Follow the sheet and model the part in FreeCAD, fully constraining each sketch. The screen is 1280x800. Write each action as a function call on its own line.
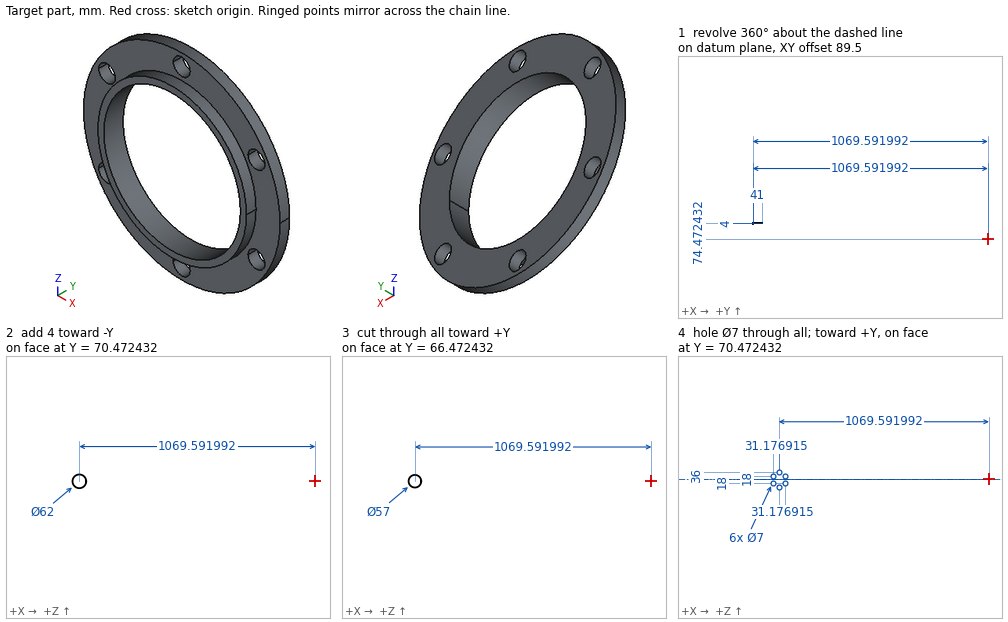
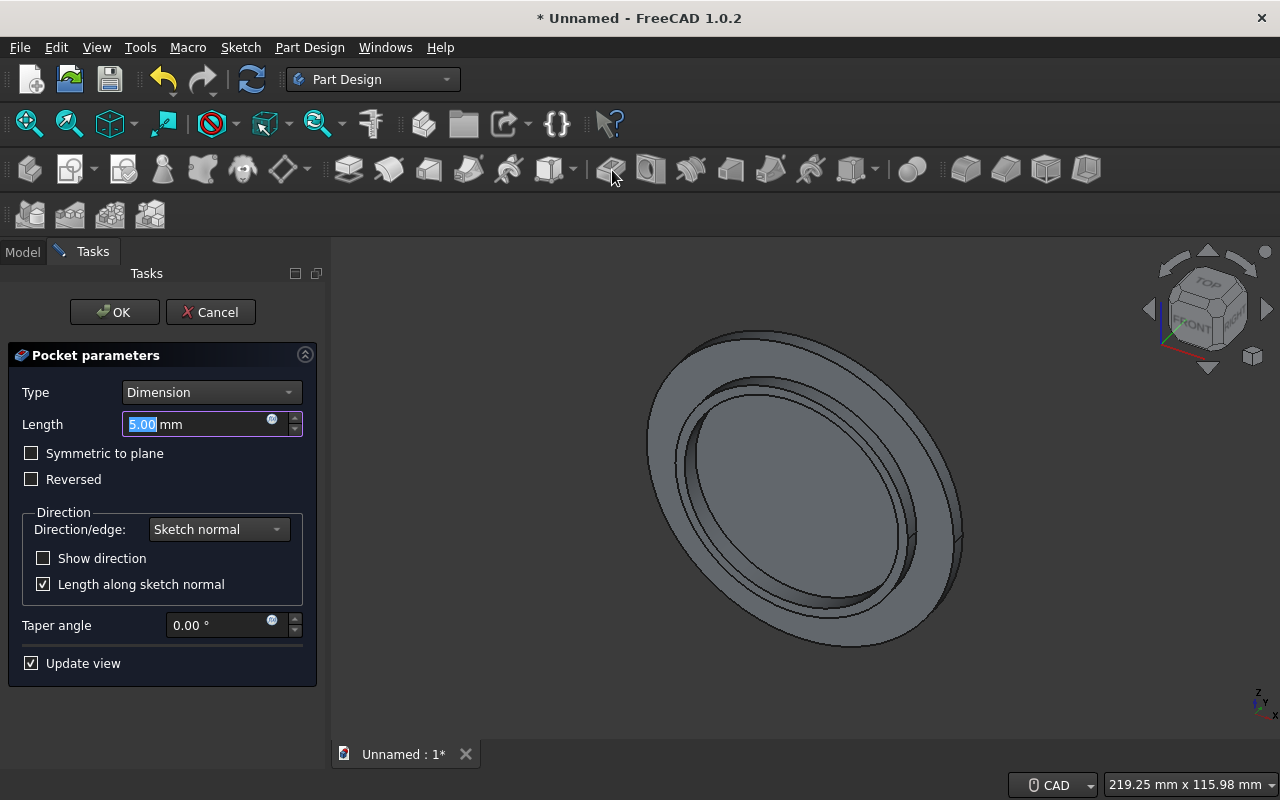
click(212, 392)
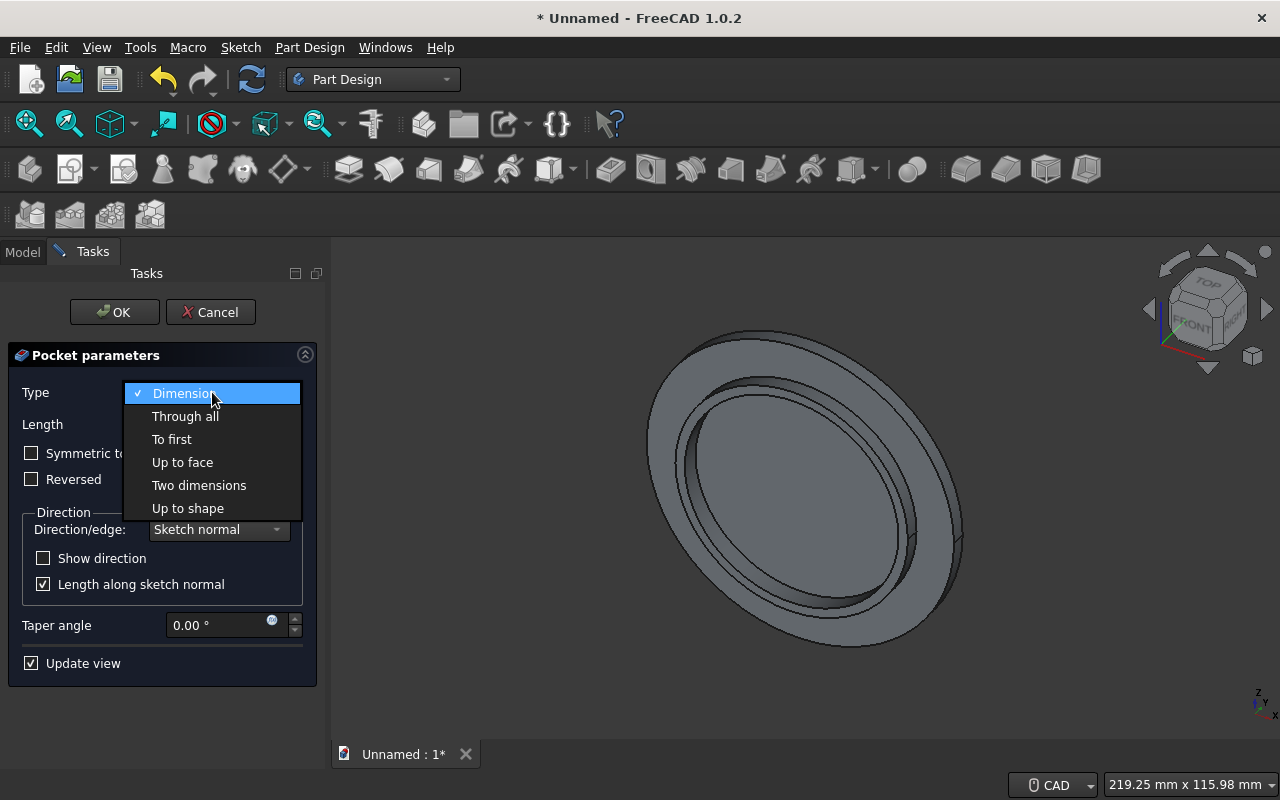
click(212, 416)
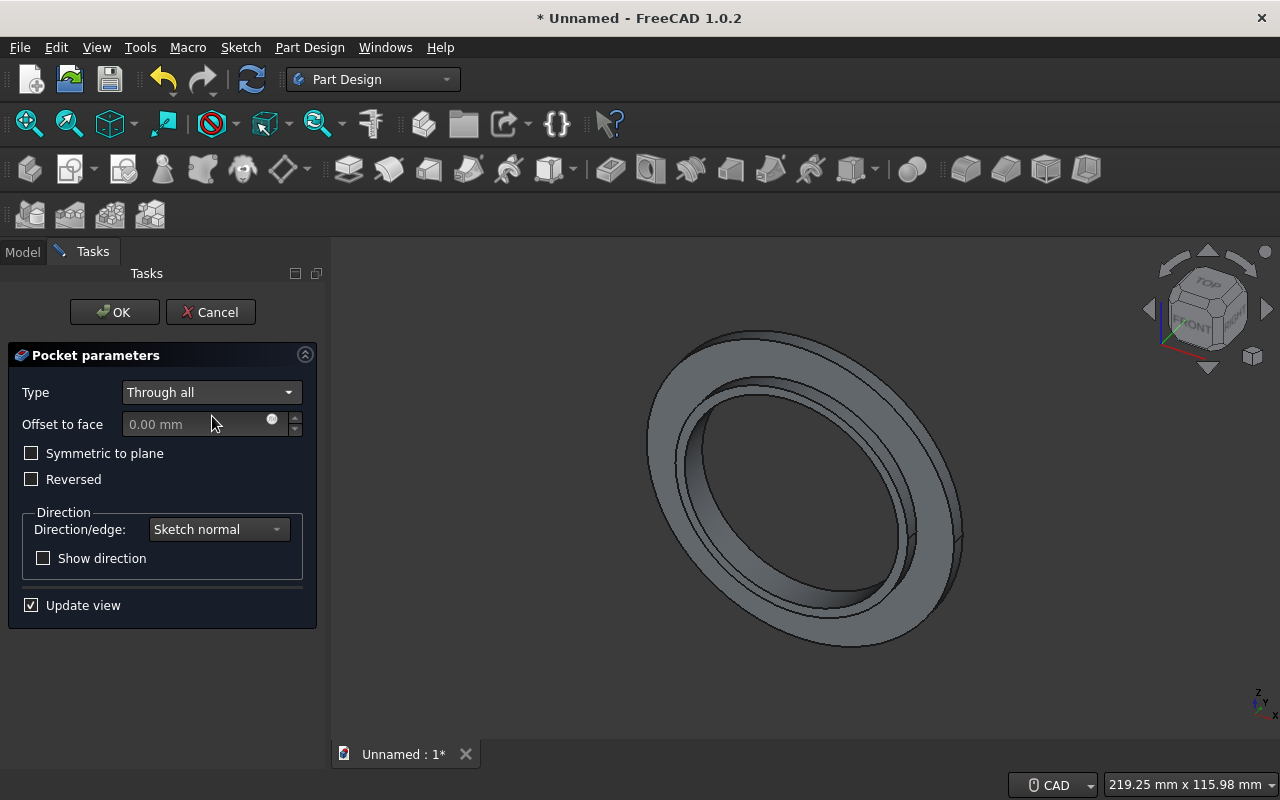
click(115, 312)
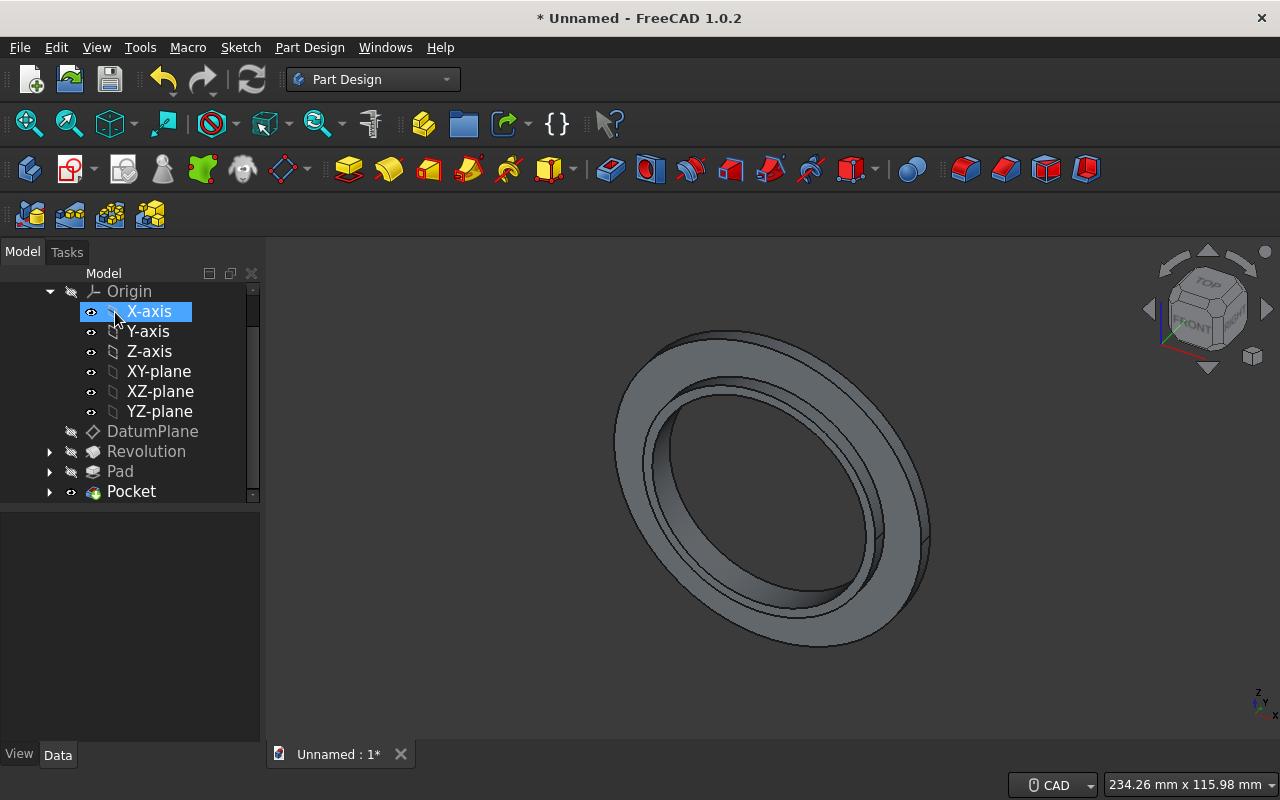
click(768, 367)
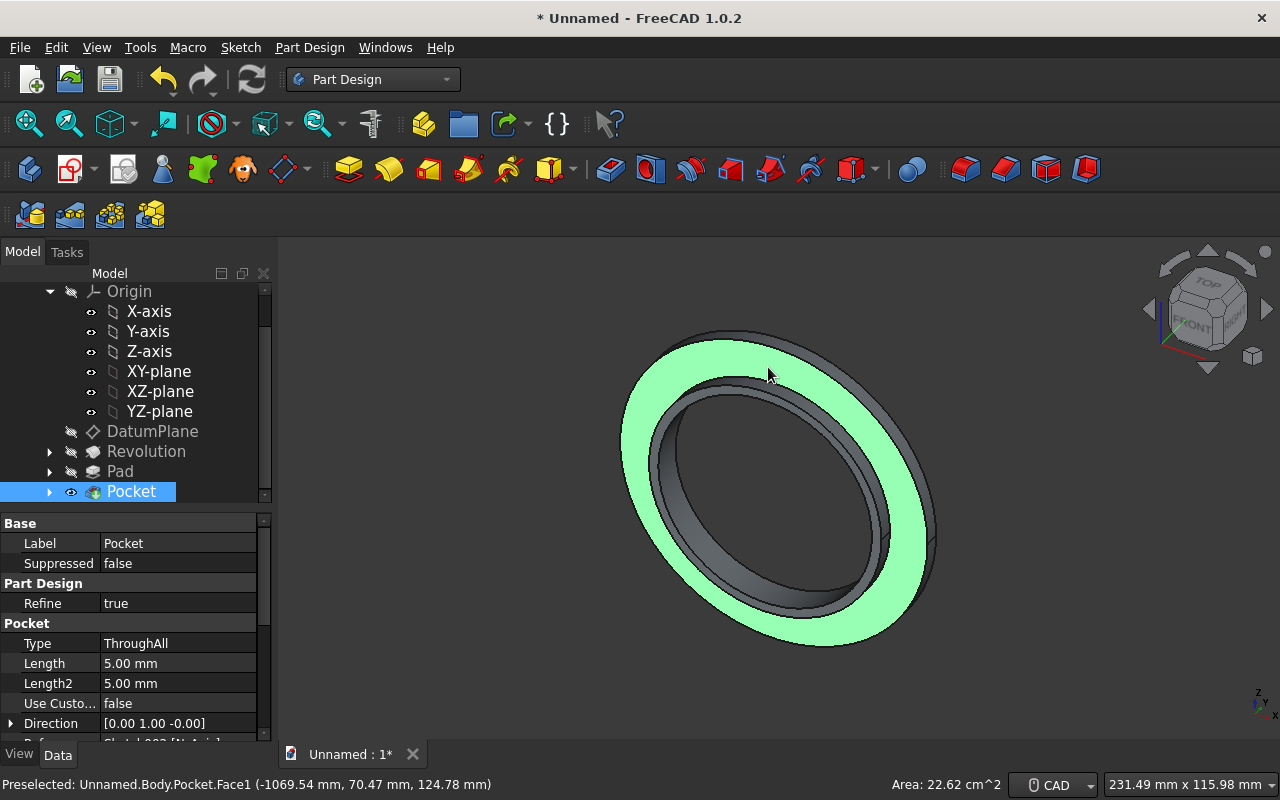
click(70, 170)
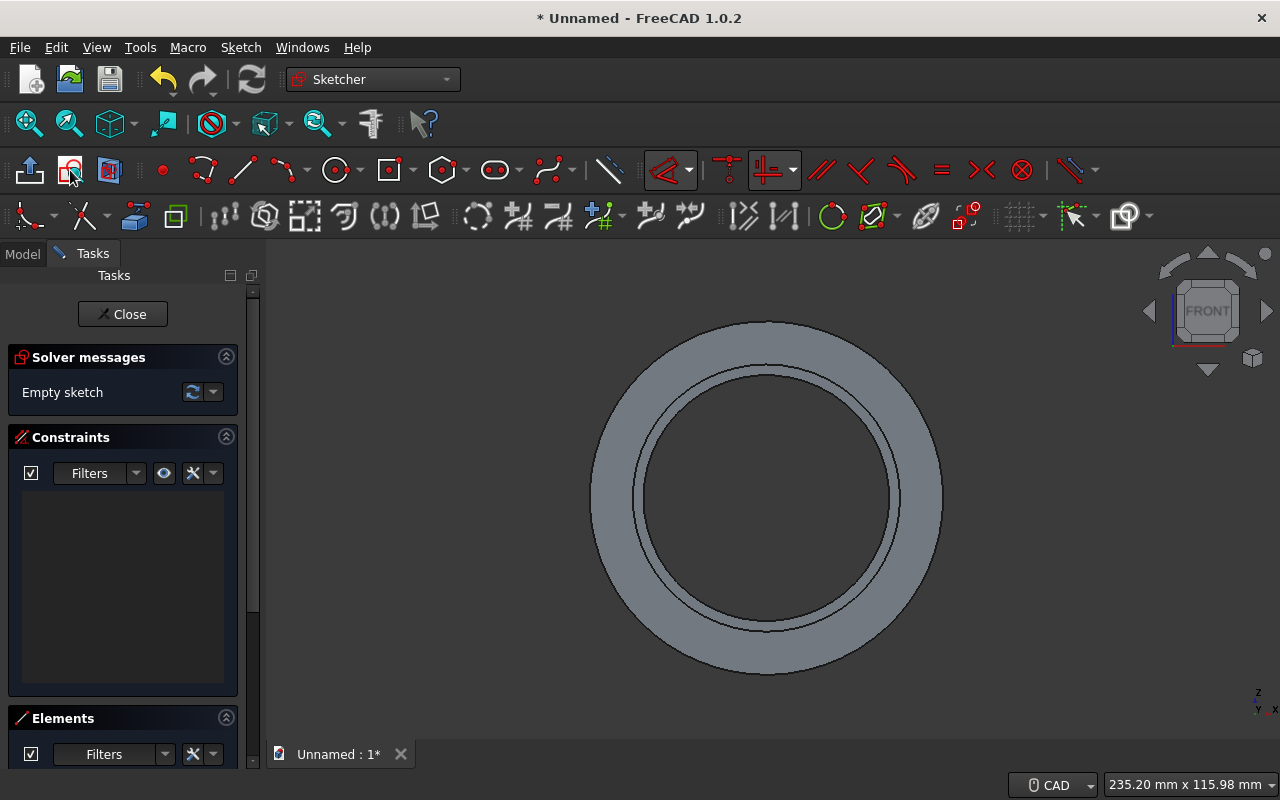
click(110, 170)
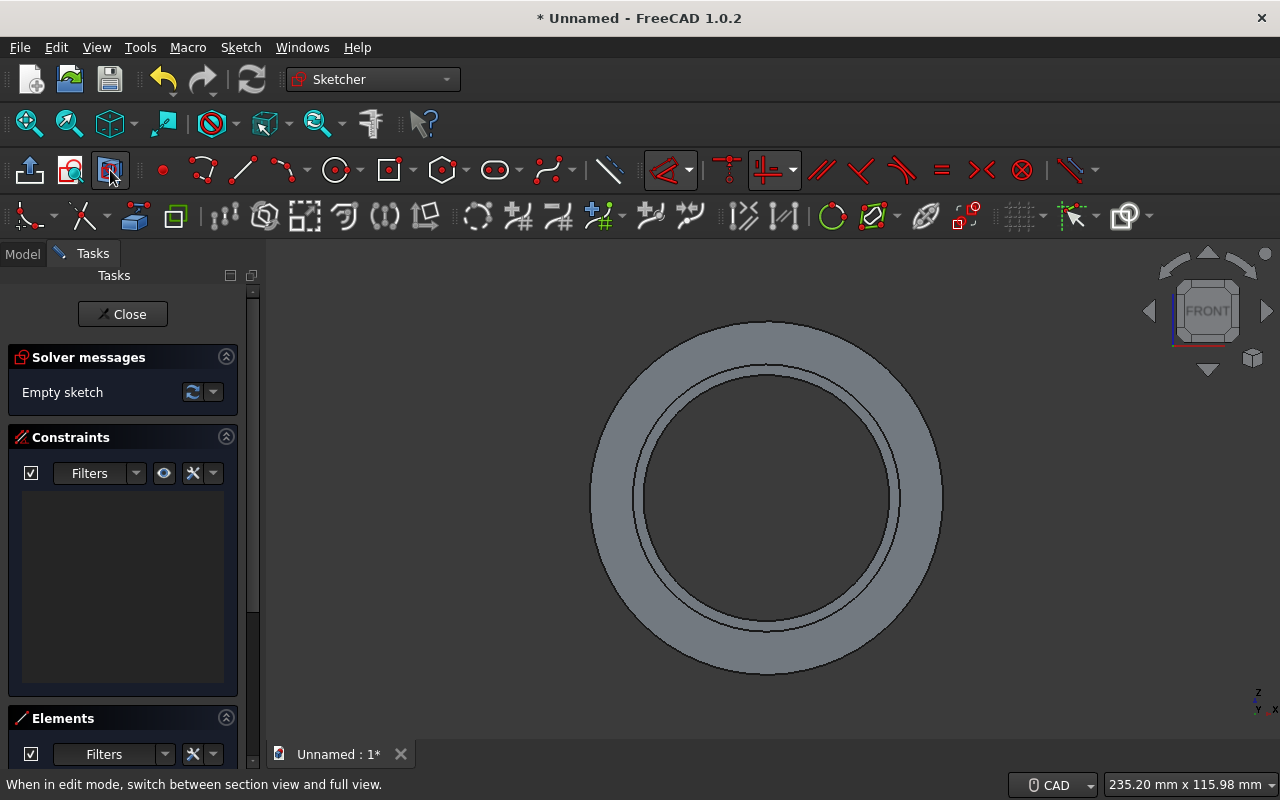
click(336, 170)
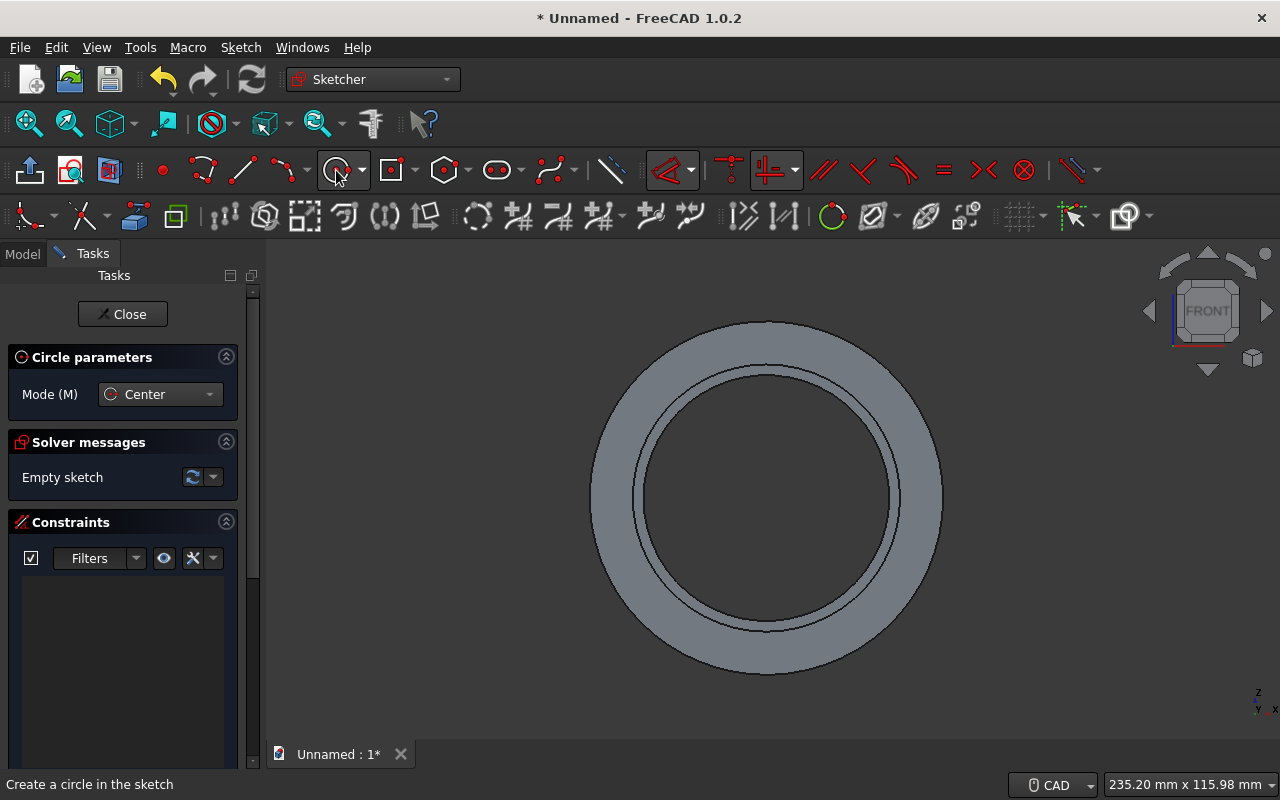
scroll(766, 343, up, 3)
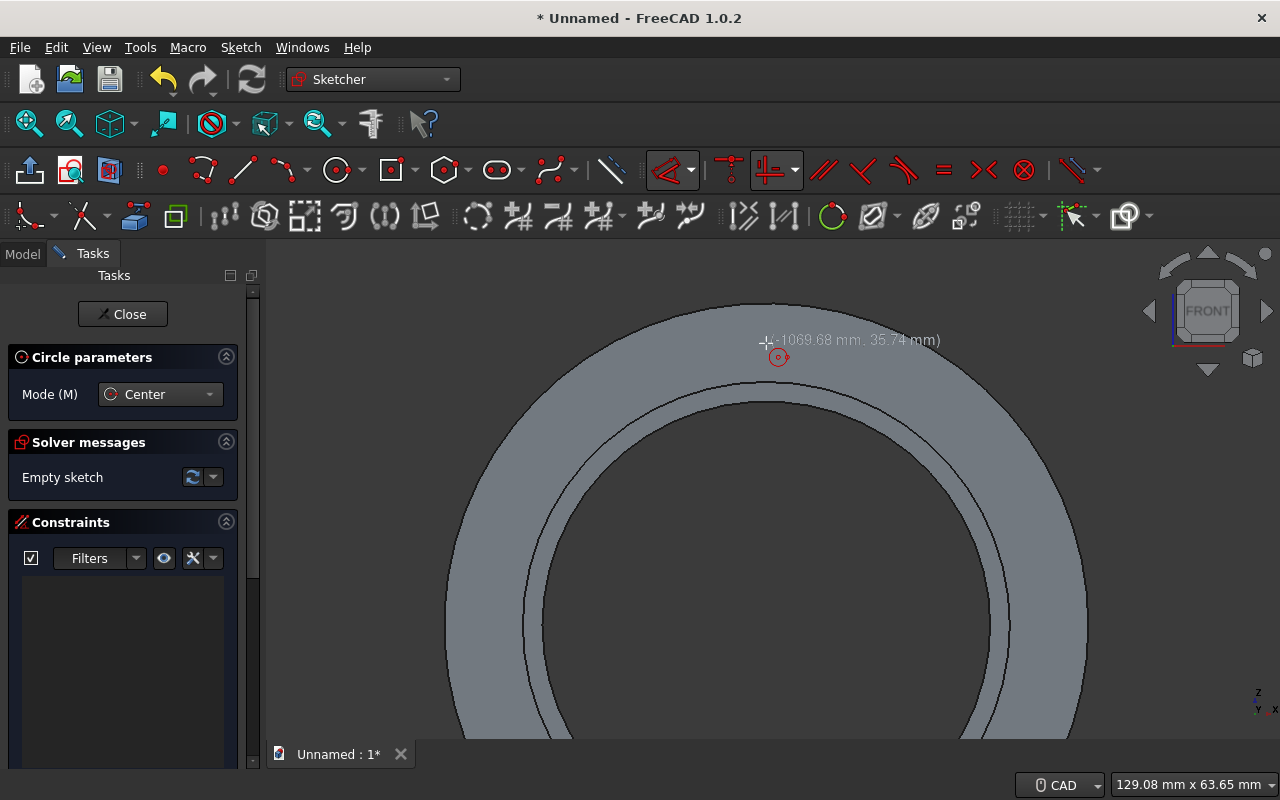
click(766, 343)
move(786, 323)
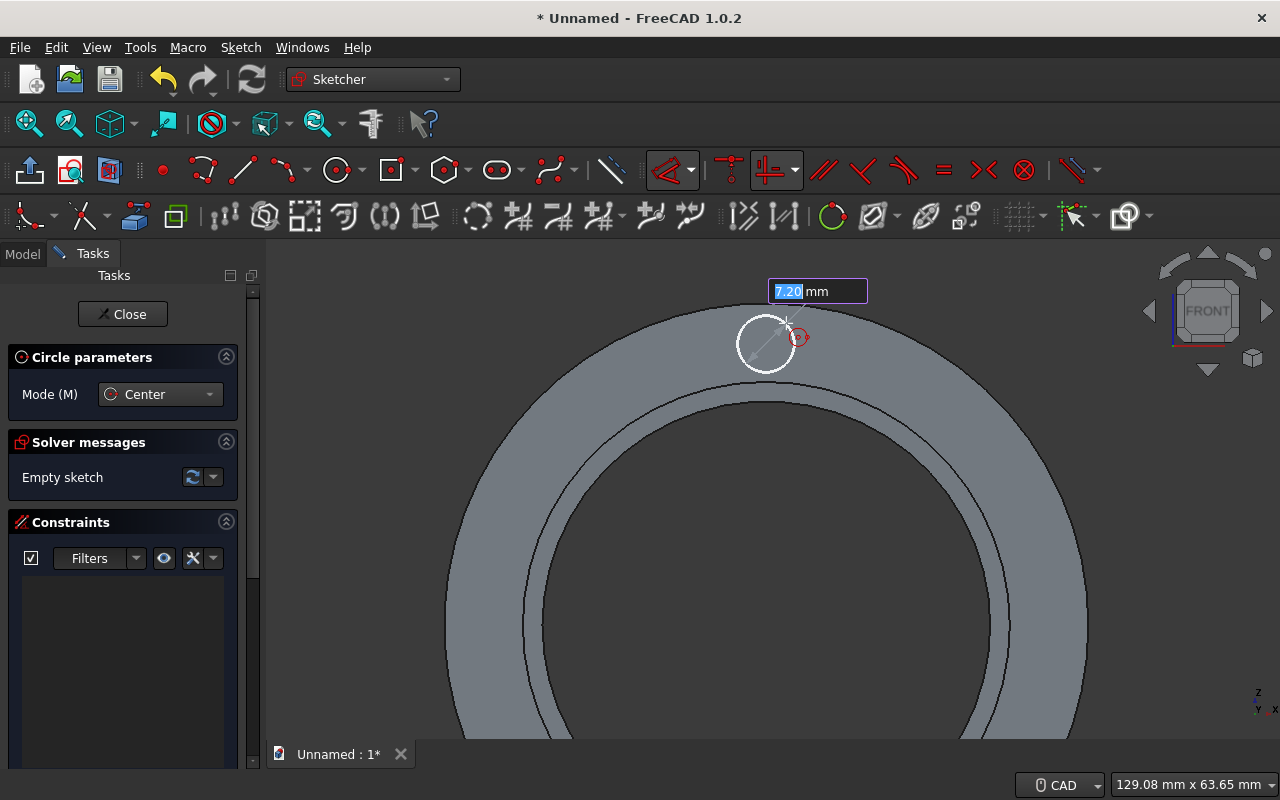
text(7)
key(Return)